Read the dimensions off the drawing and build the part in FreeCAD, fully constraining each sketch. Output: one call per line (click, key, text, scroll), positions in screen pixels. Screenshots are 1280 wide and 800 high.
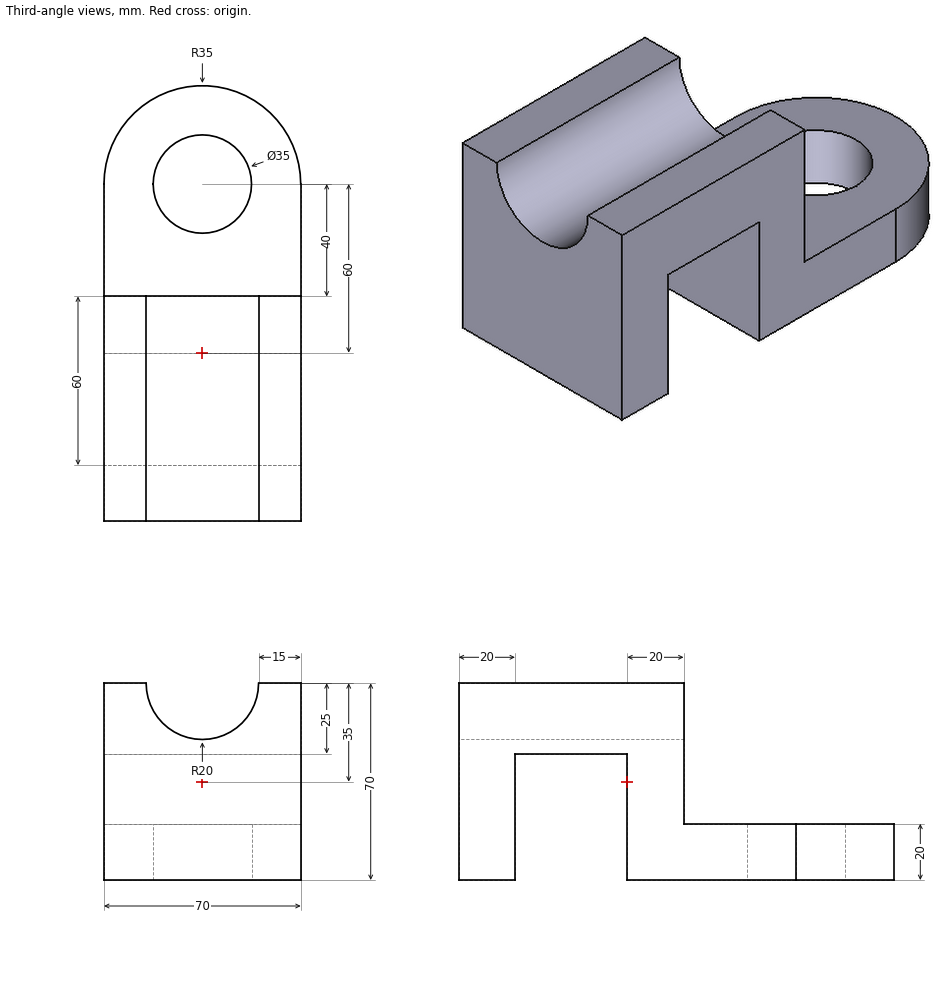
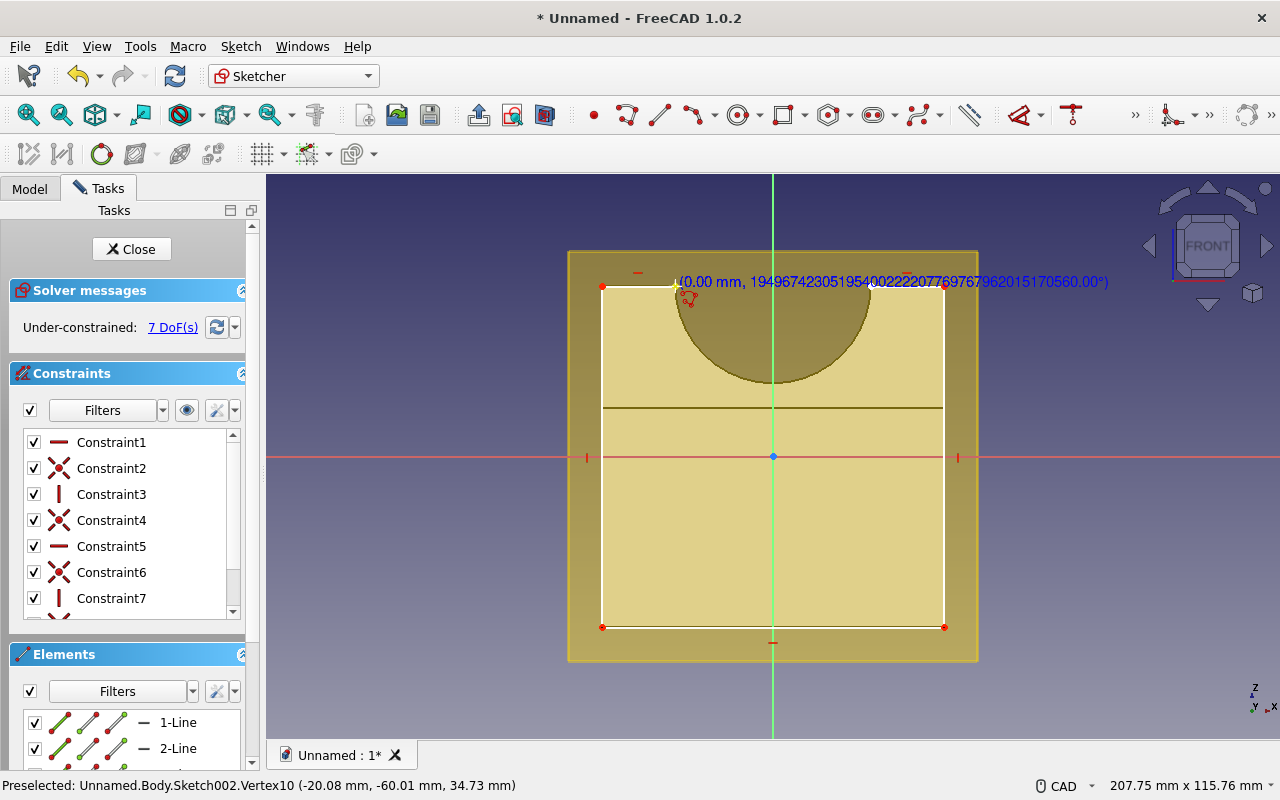
click(692, 116)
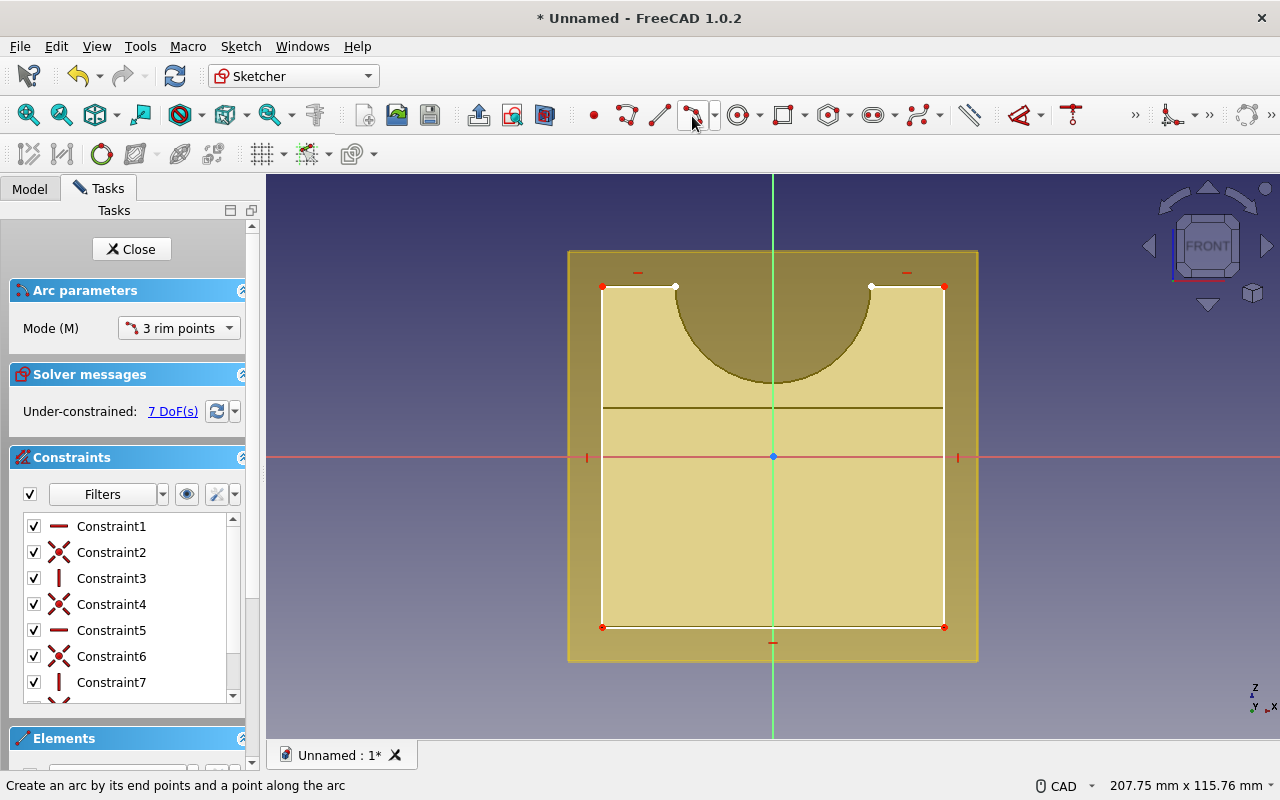
click(675, 287)
click(871, 287)
click(743, 379)
key(Escape)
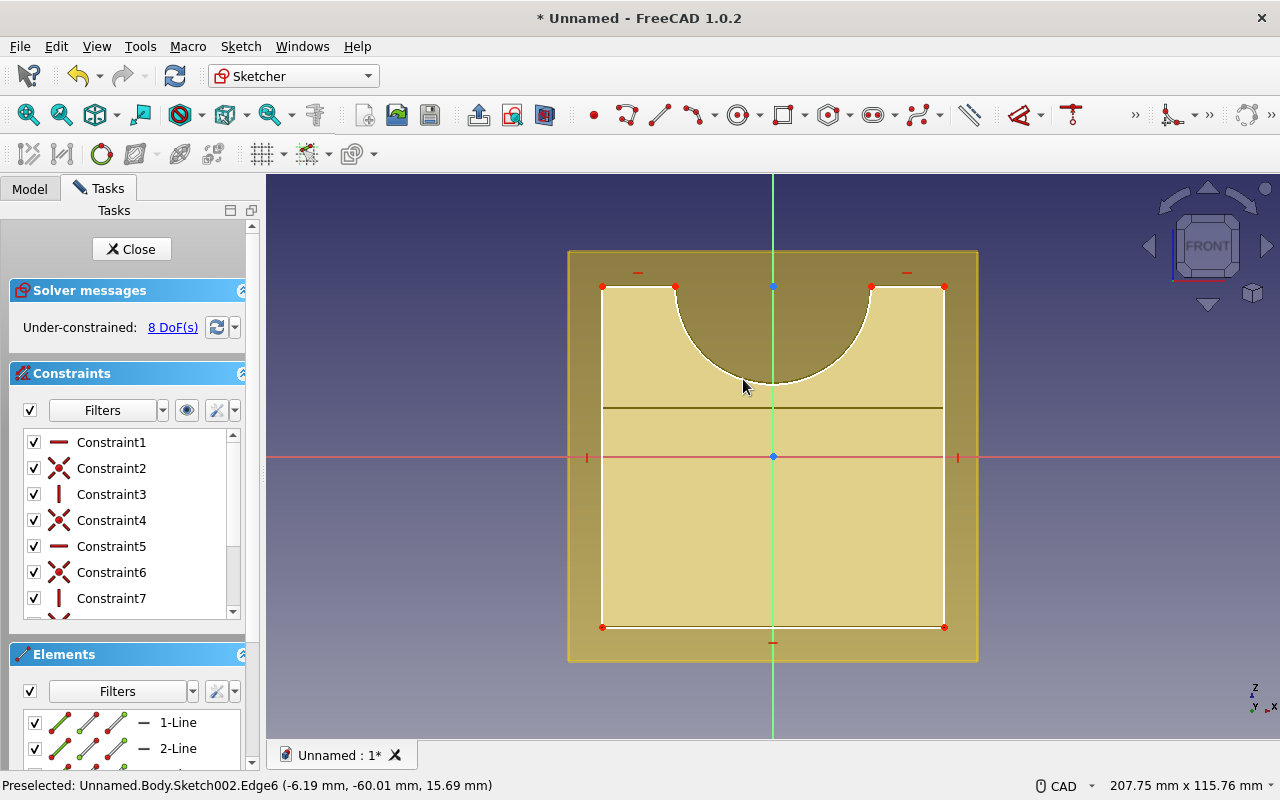
click(773, 287)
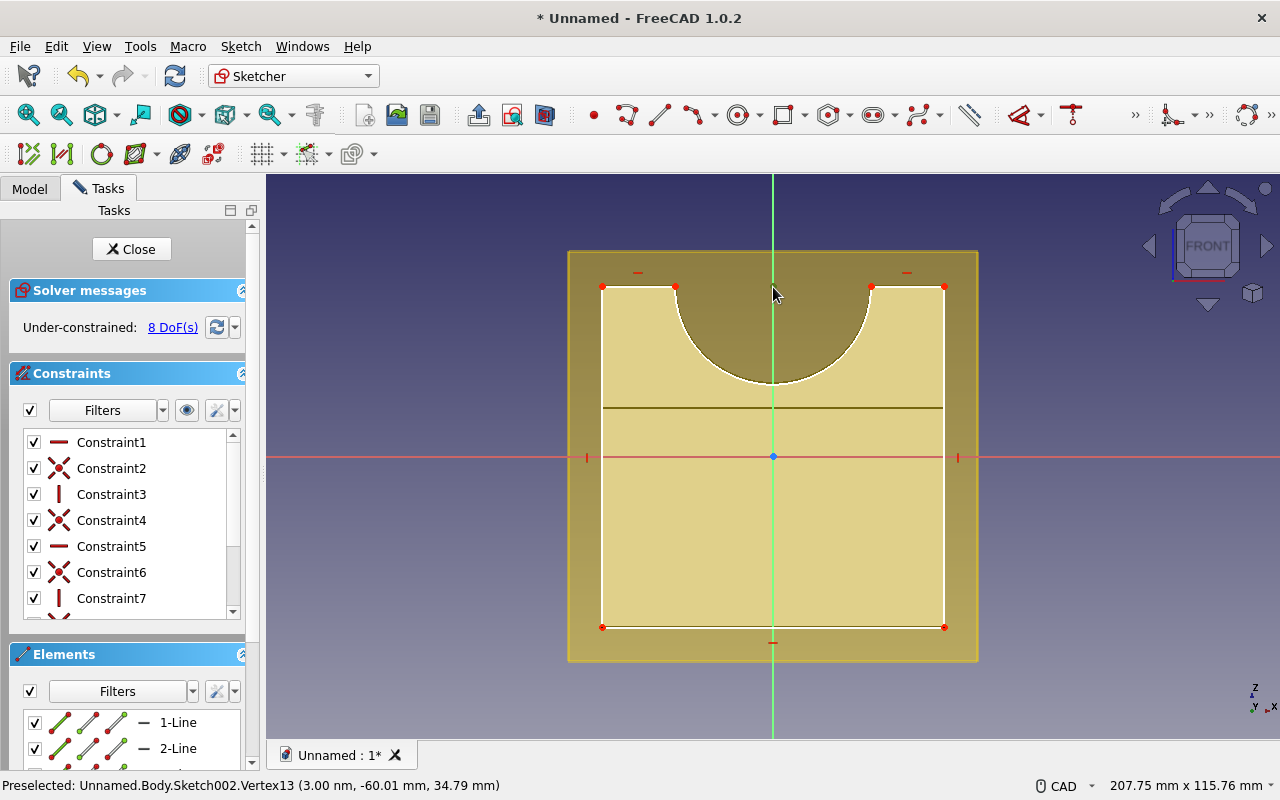
click(773, 675)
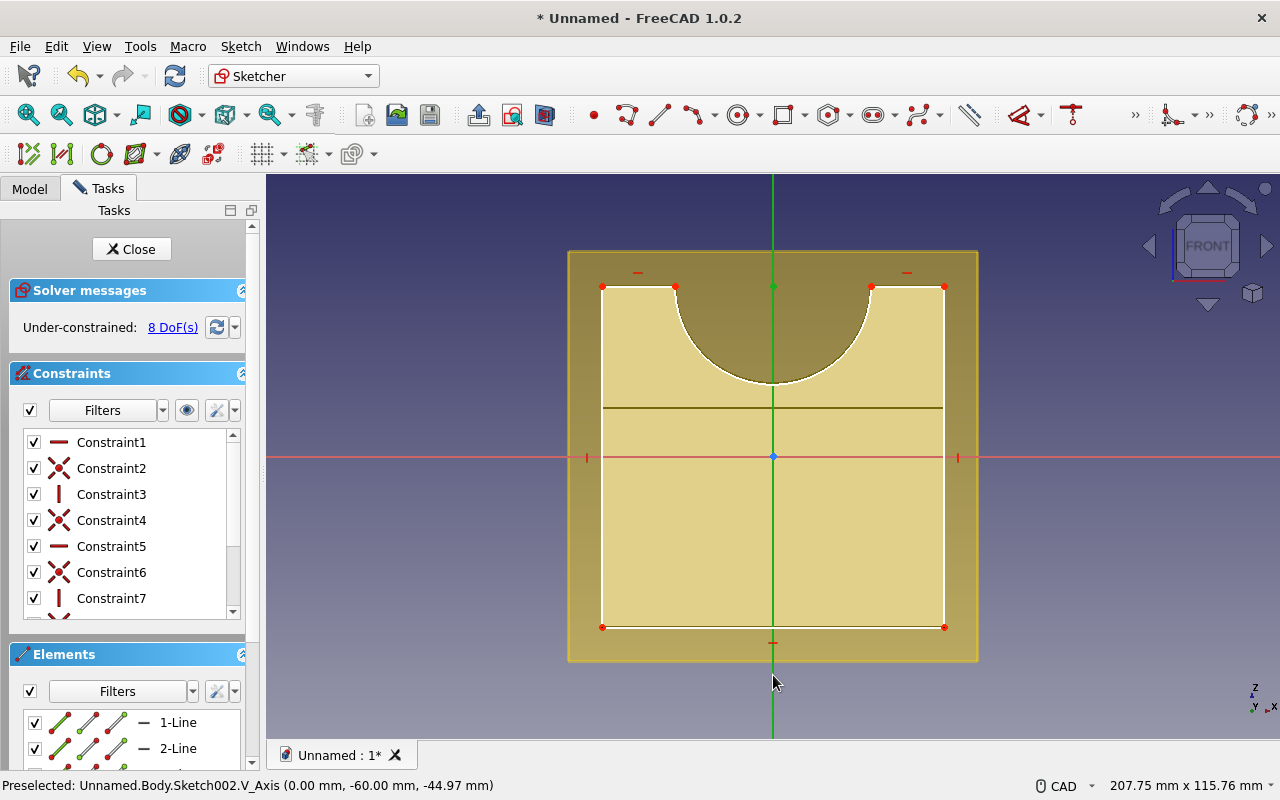
click(1071, 116)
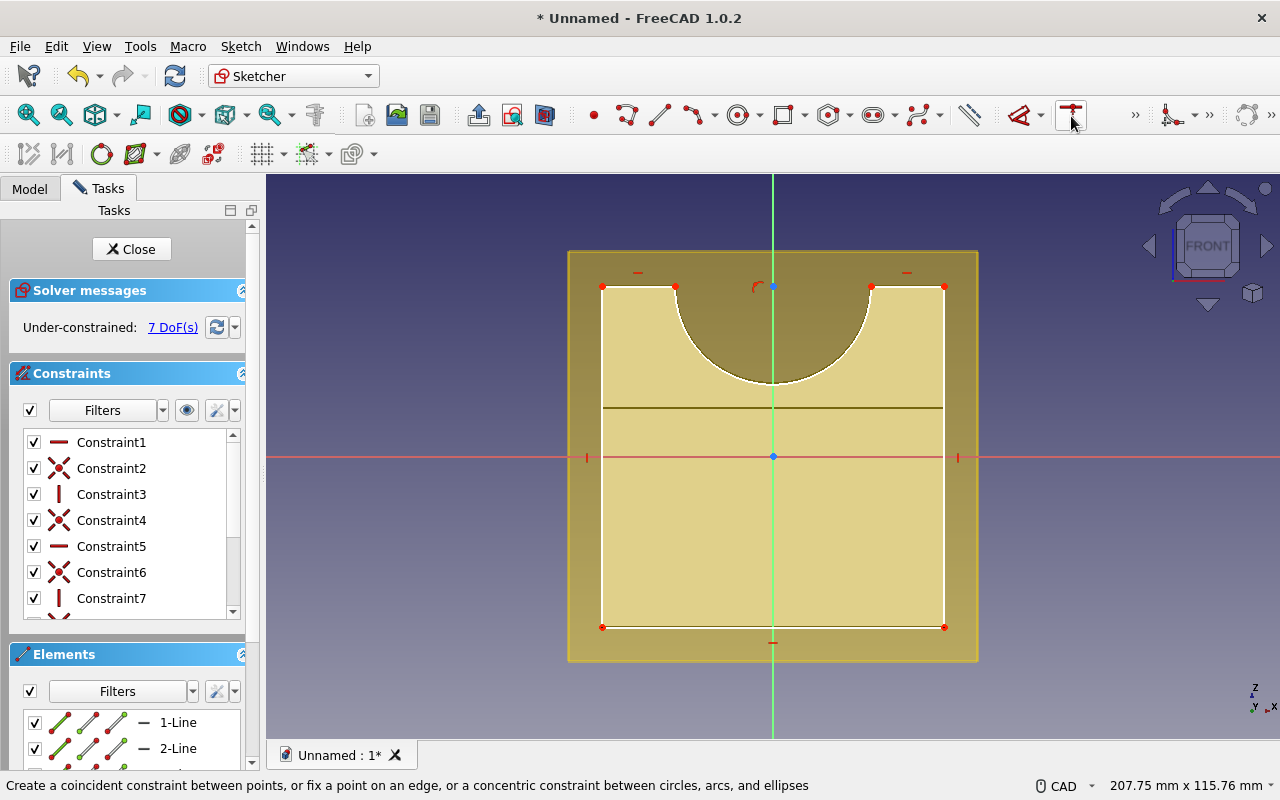
click(1018, 116)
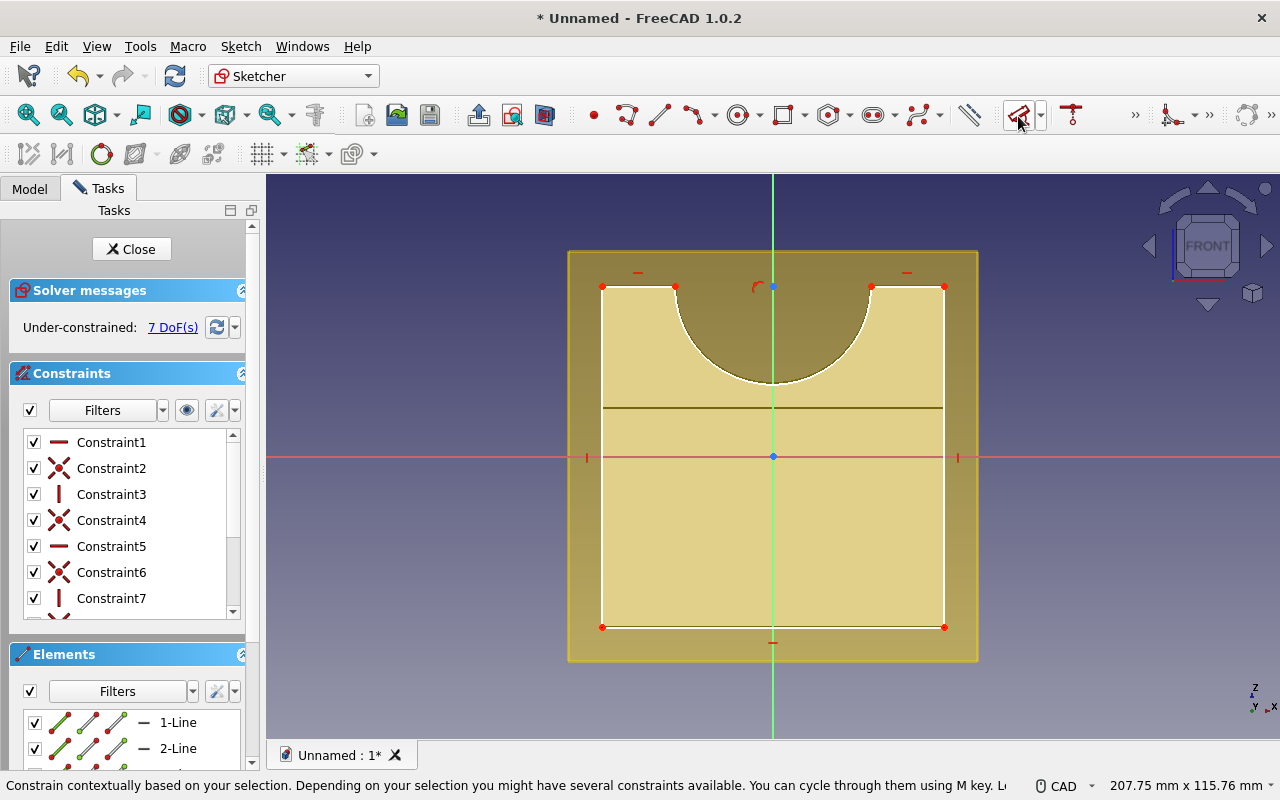
click(715, 366)
click(696, 392)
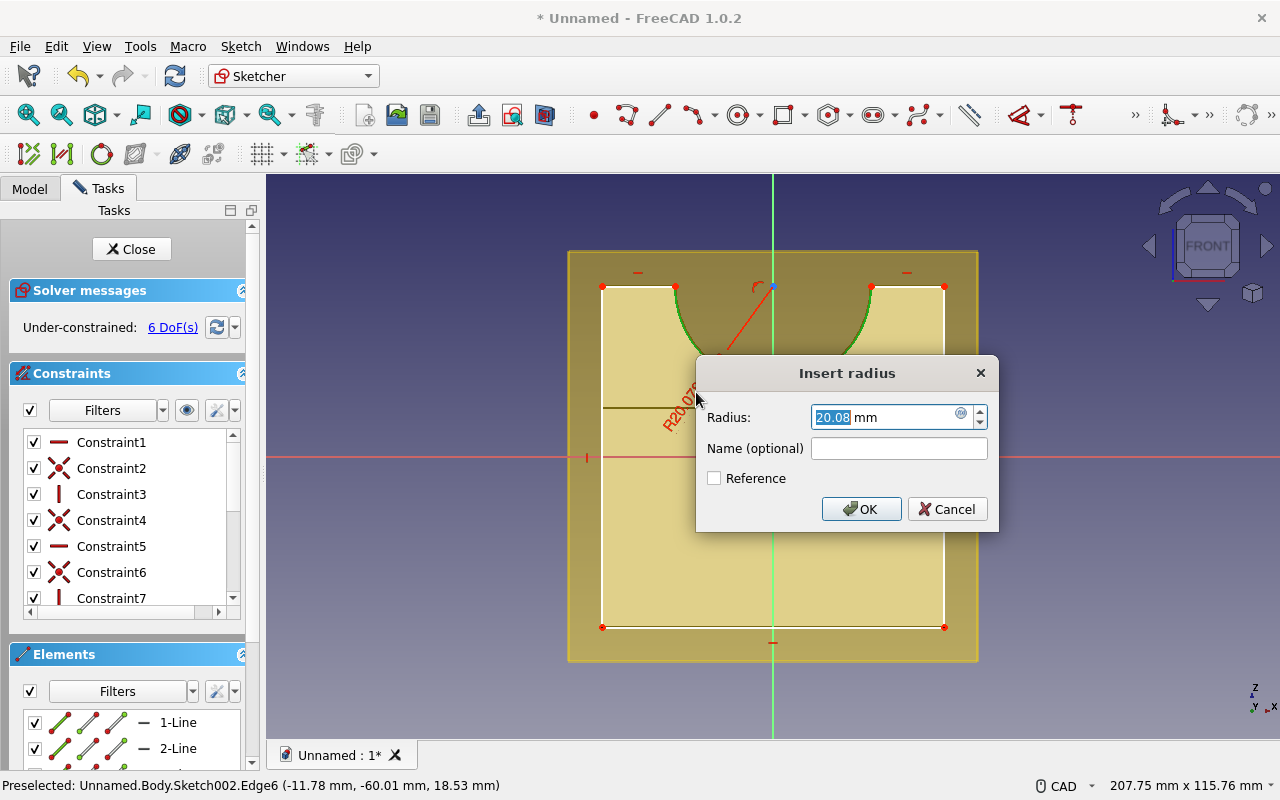
text(20)
key(Return)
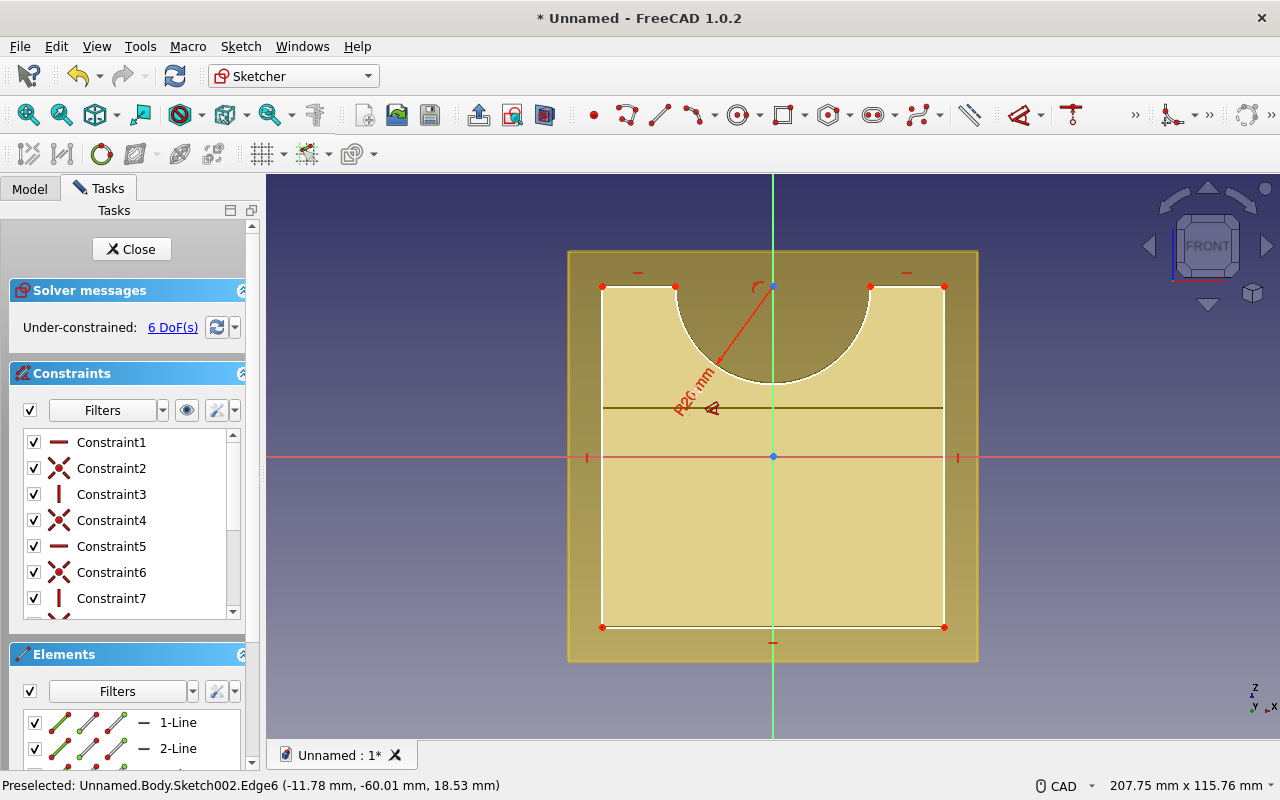
click(893, 287)
click(907, 253)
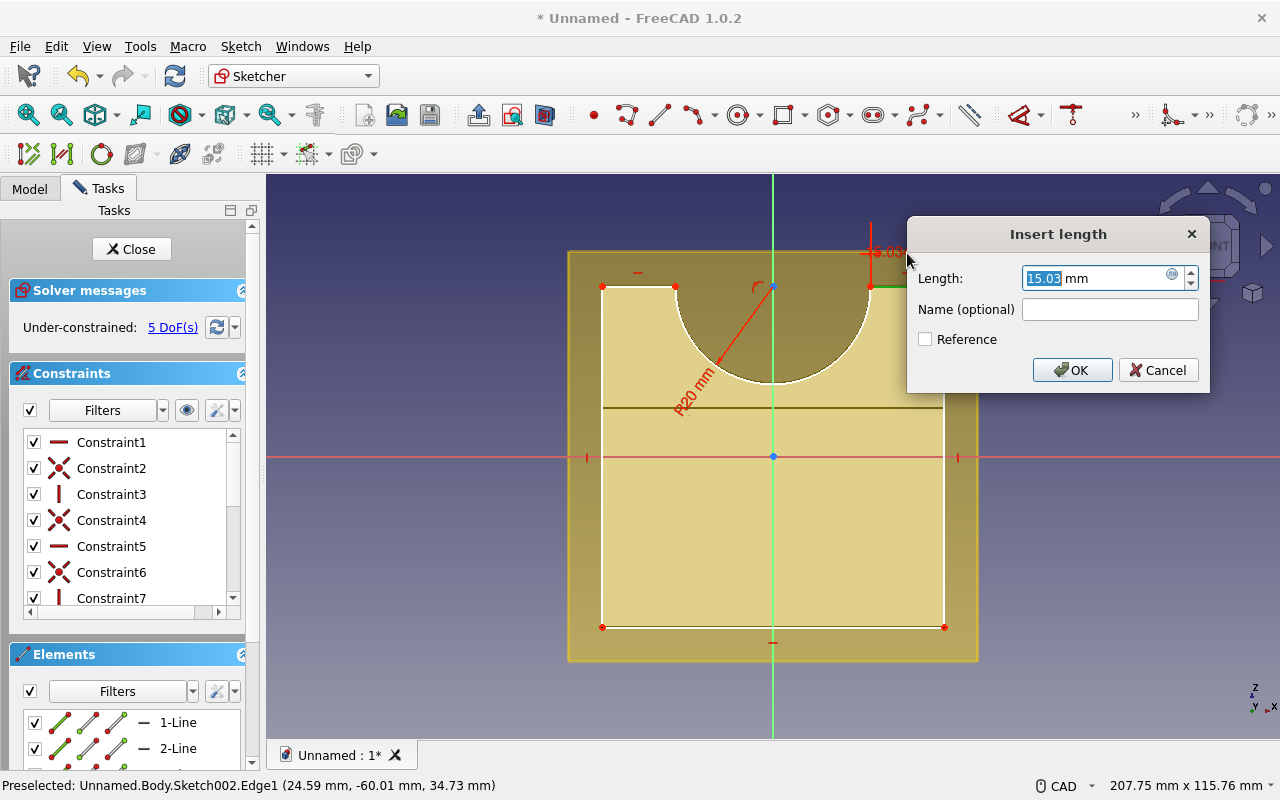
text(15)
key(Return)